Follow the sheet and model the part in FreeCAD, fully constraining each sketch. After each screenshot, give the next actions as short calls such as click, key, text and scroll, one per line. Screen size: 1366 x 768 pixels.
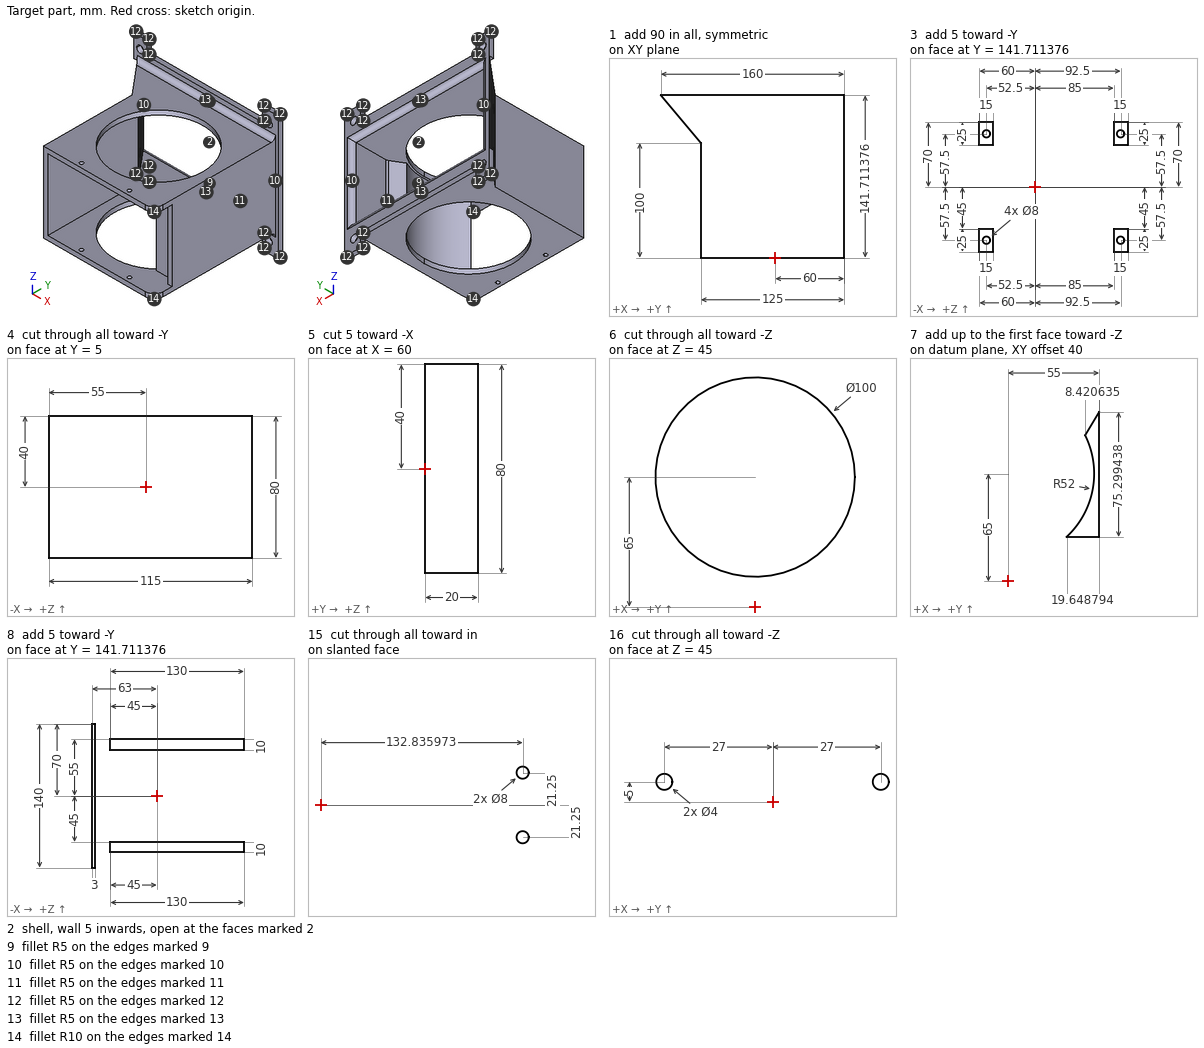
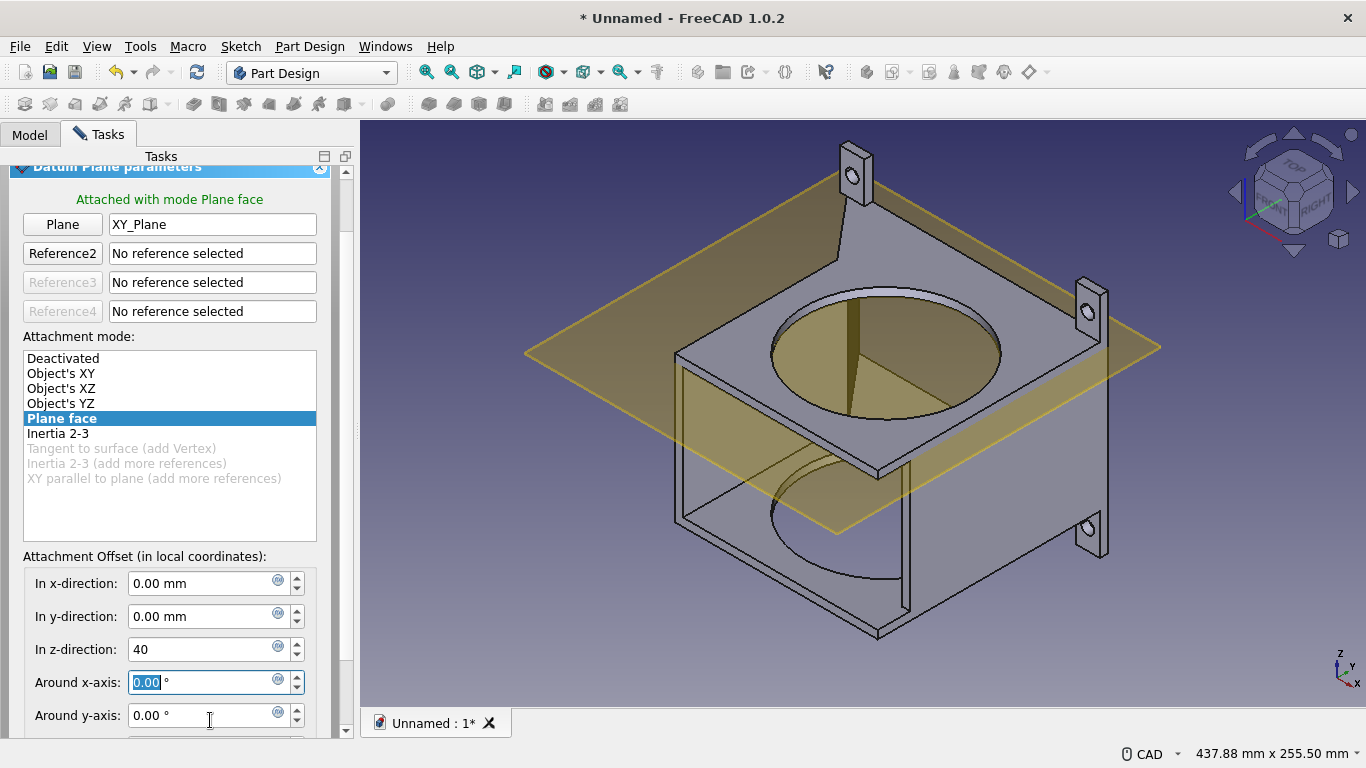
scroll(346, 452, up, 2)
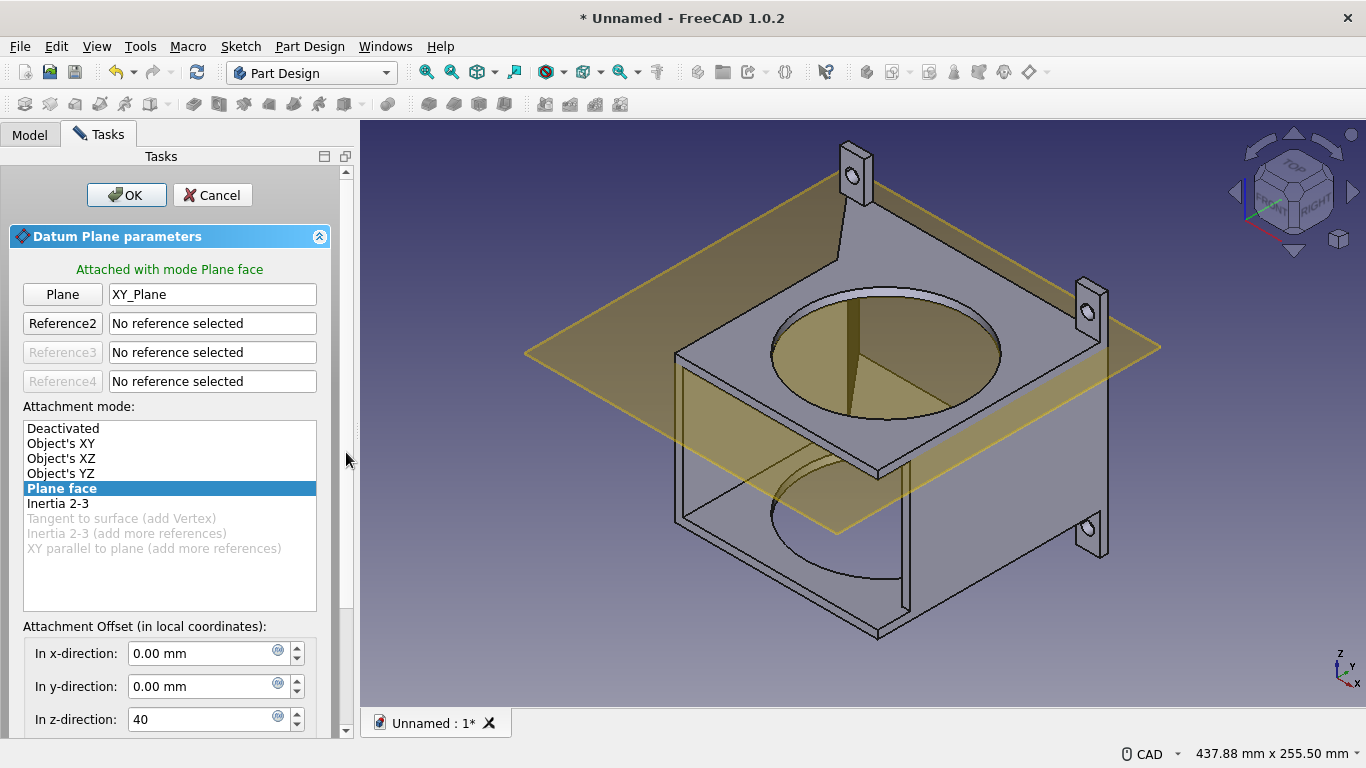
click(127, 195)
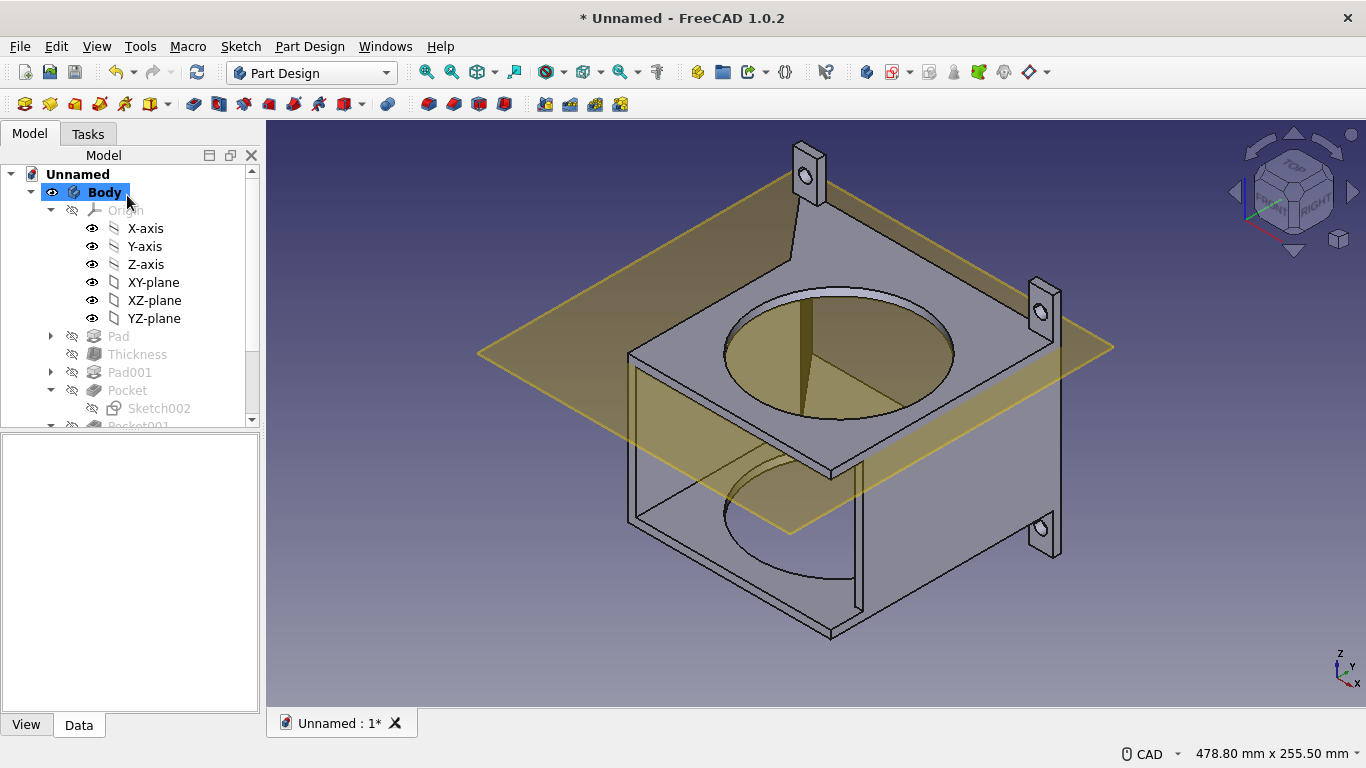
scroll(101, 296, down, 3)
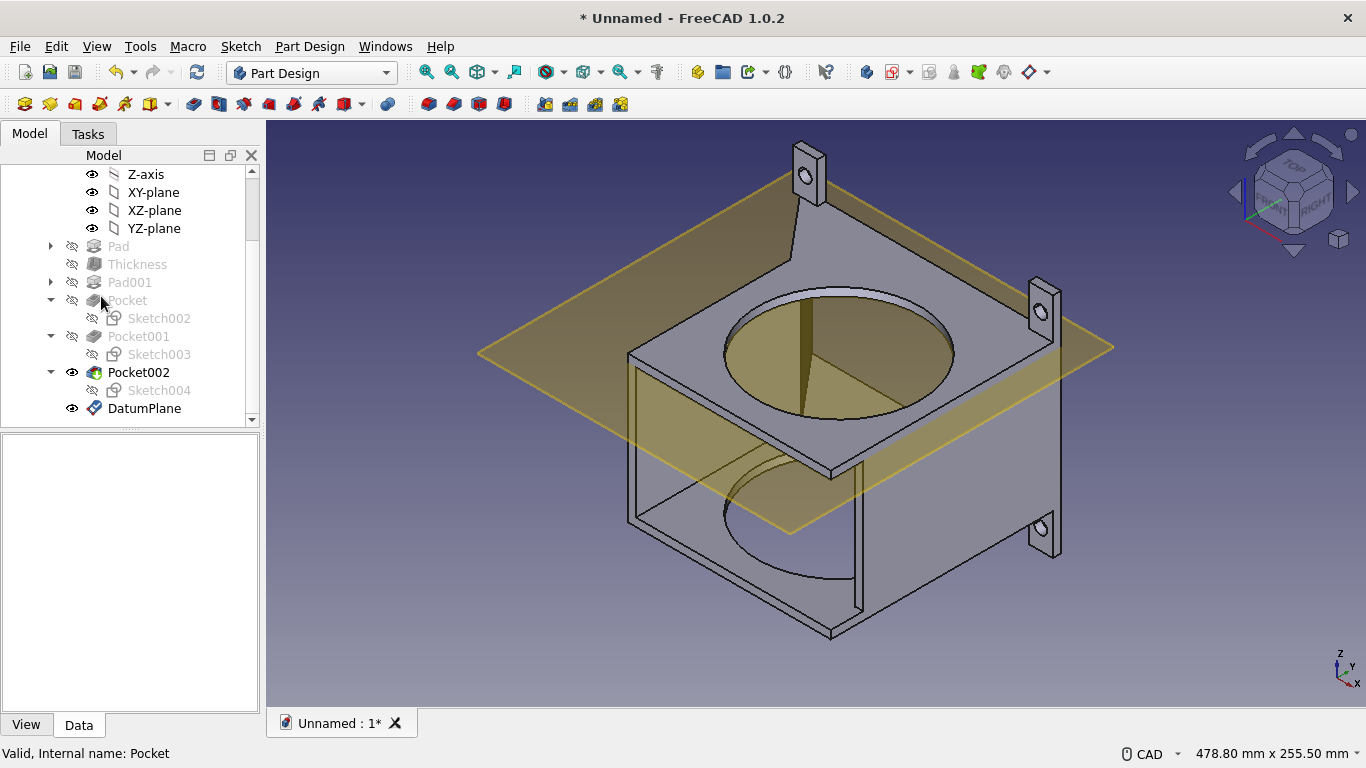
click(117, 408)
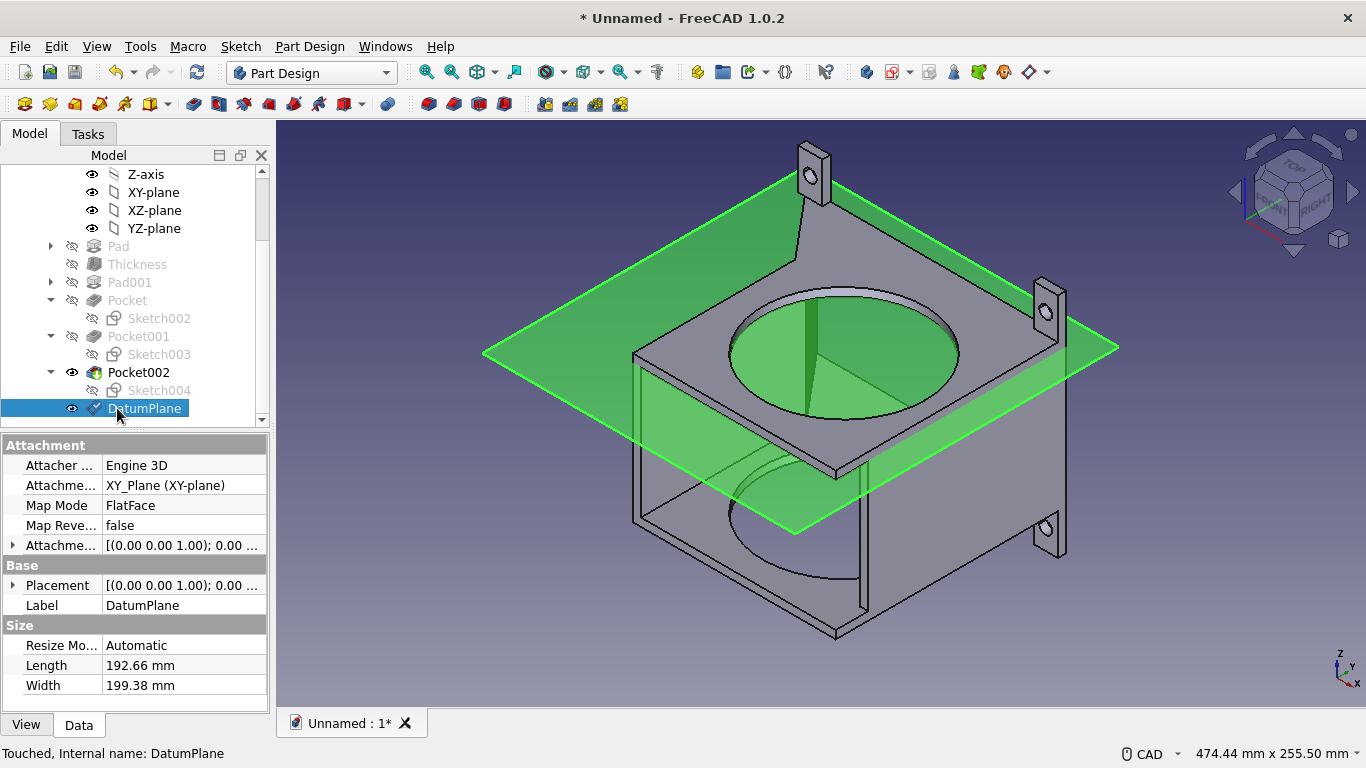
click(892, 72)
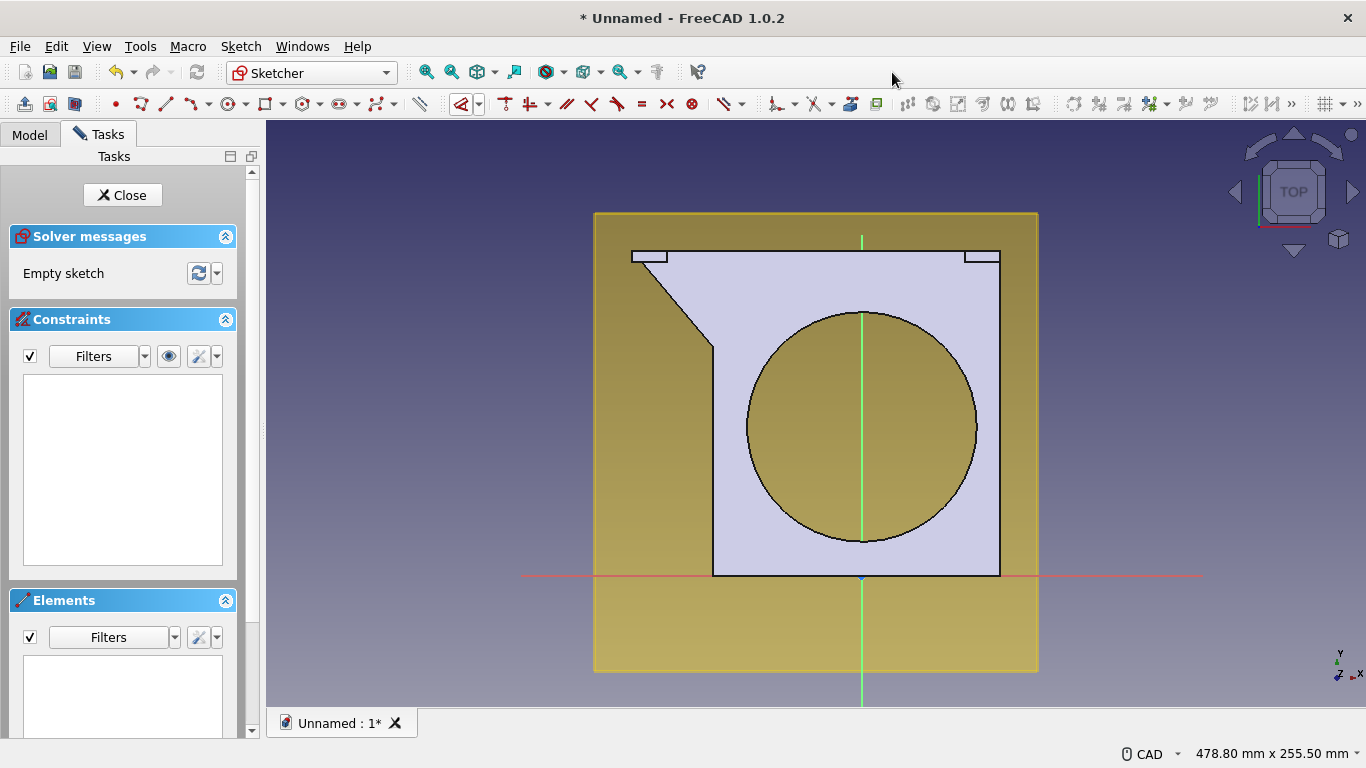
key(q)
key(s)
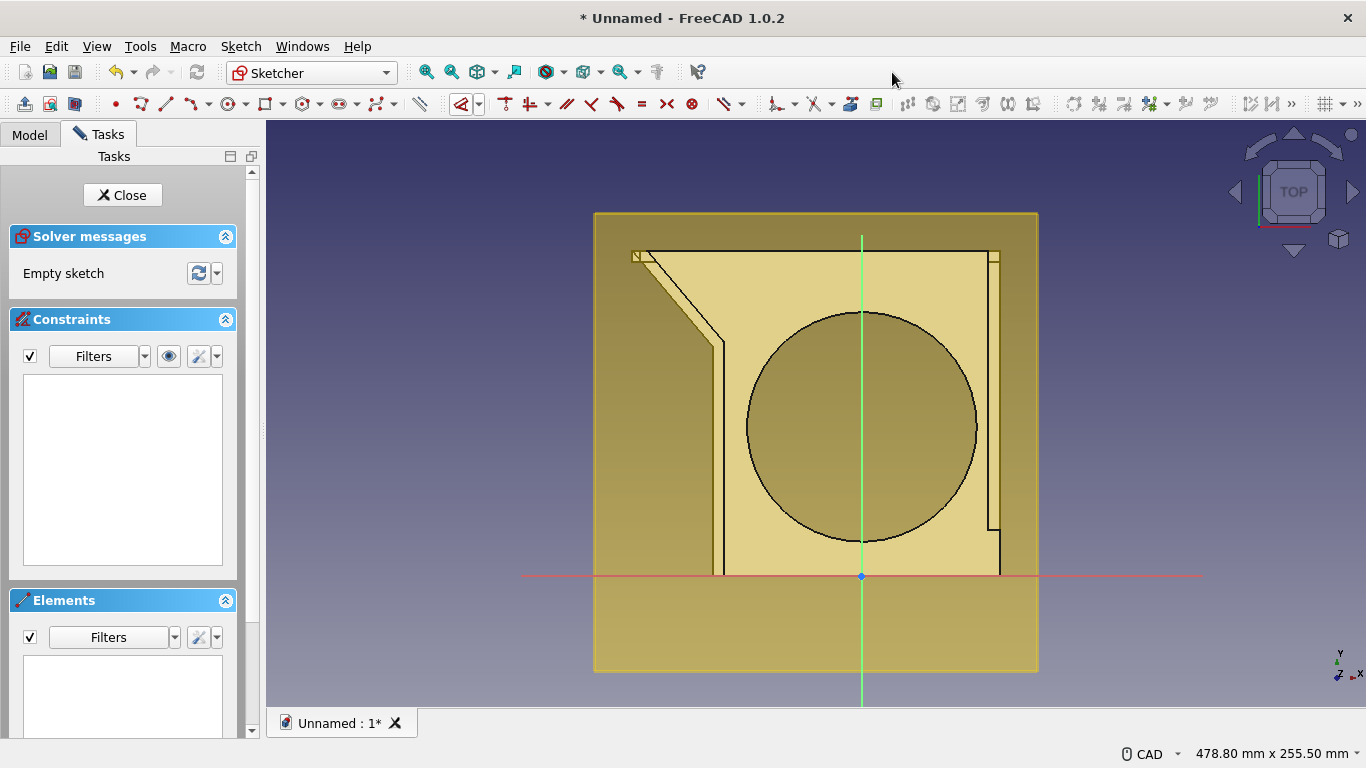
scroll(1201, 551, up, 2)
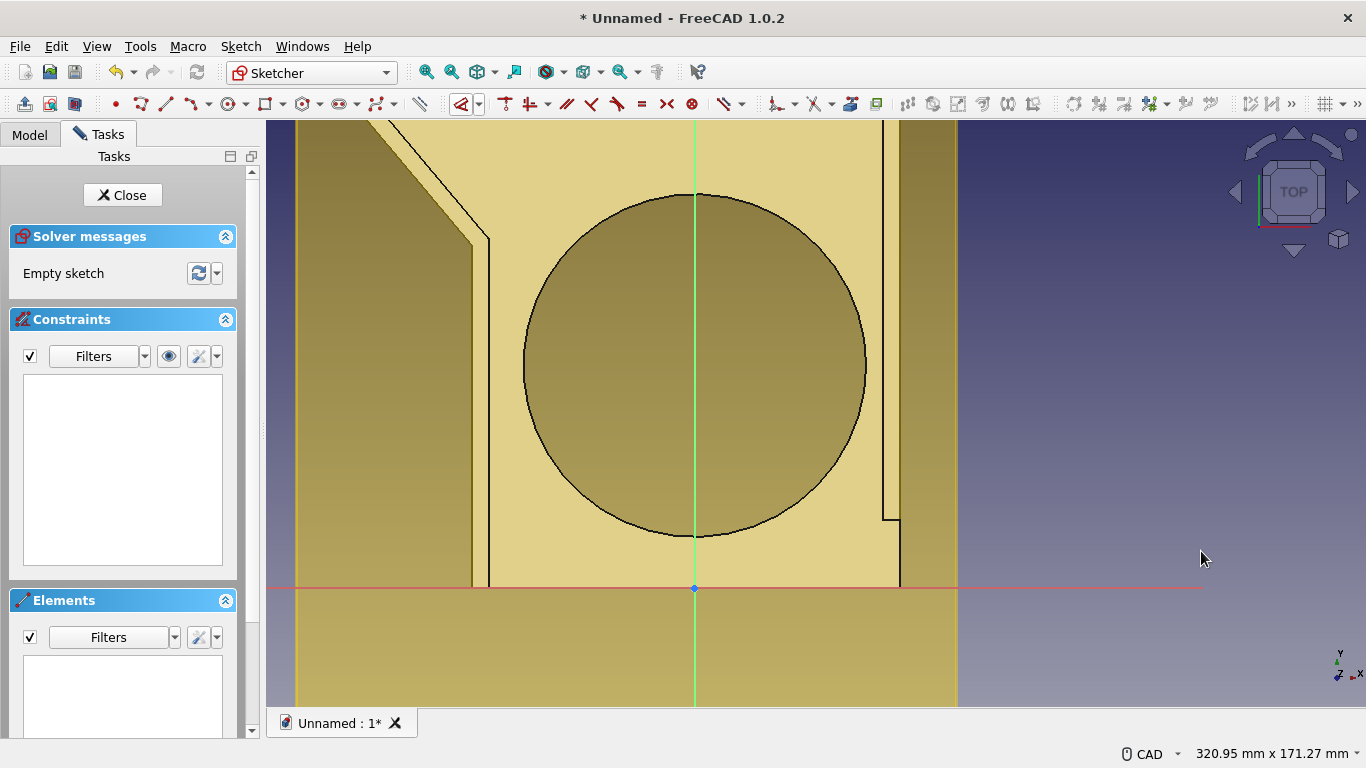
click(141, 104)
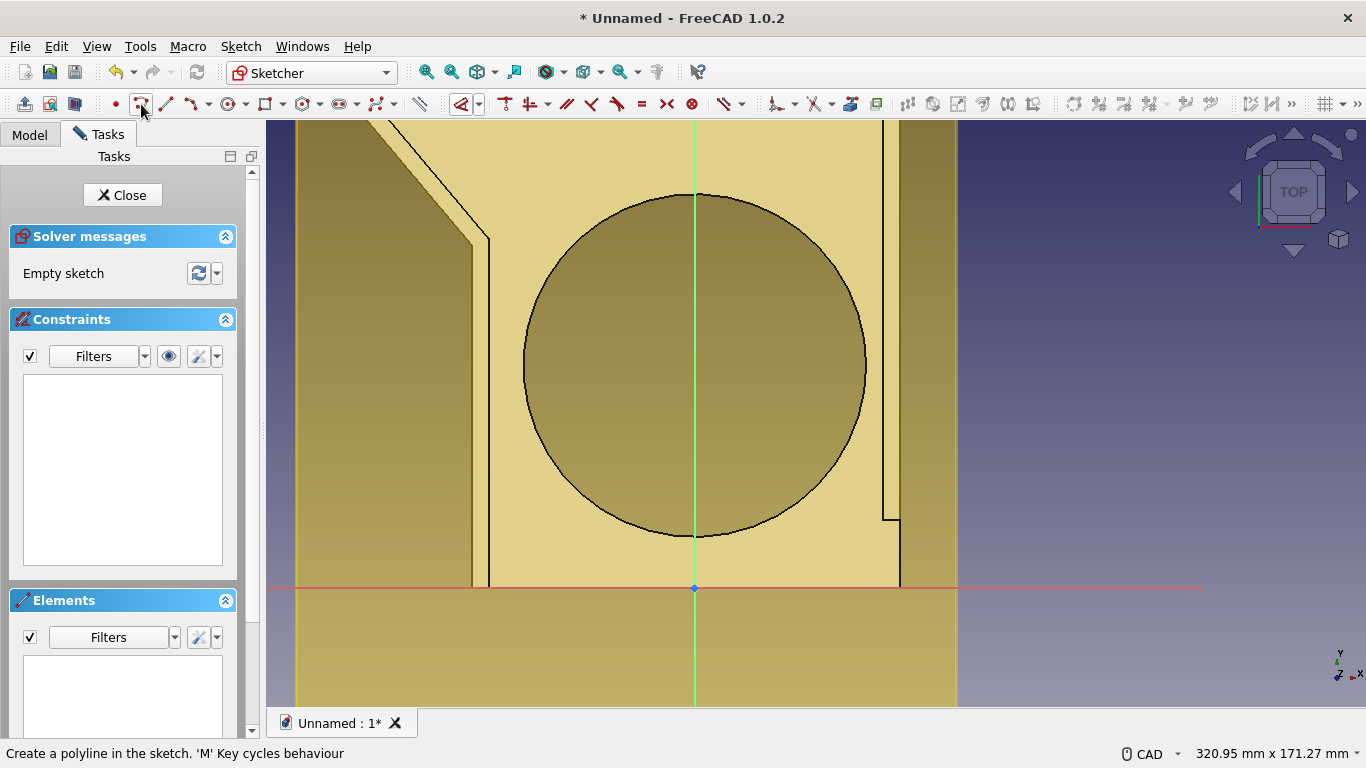
click(854, 286)
click(883, 238)
click(883, 496)
click(816, 496)
right_click(816, 496)